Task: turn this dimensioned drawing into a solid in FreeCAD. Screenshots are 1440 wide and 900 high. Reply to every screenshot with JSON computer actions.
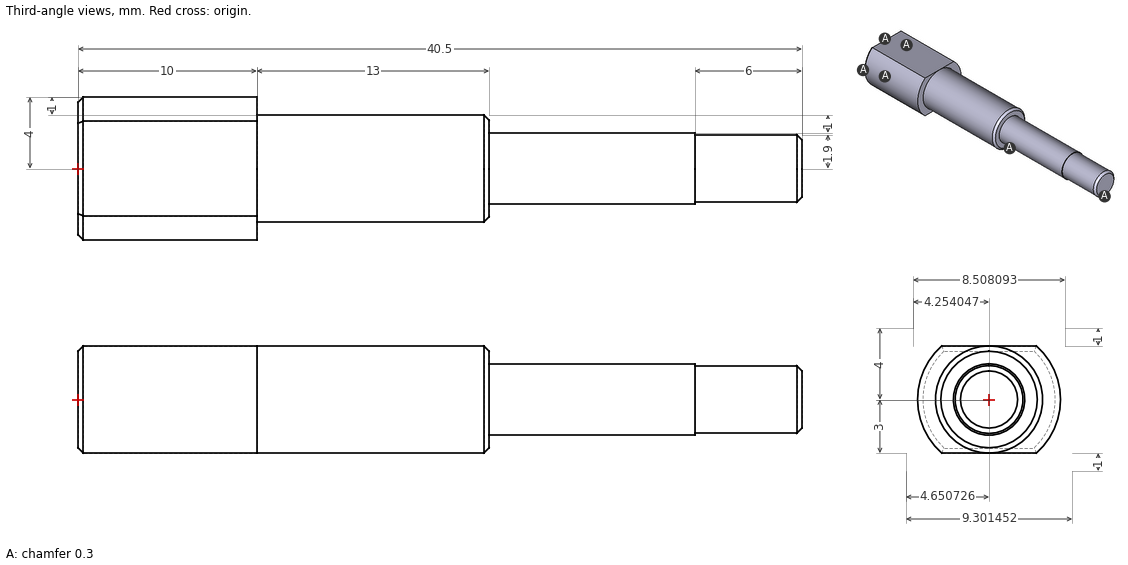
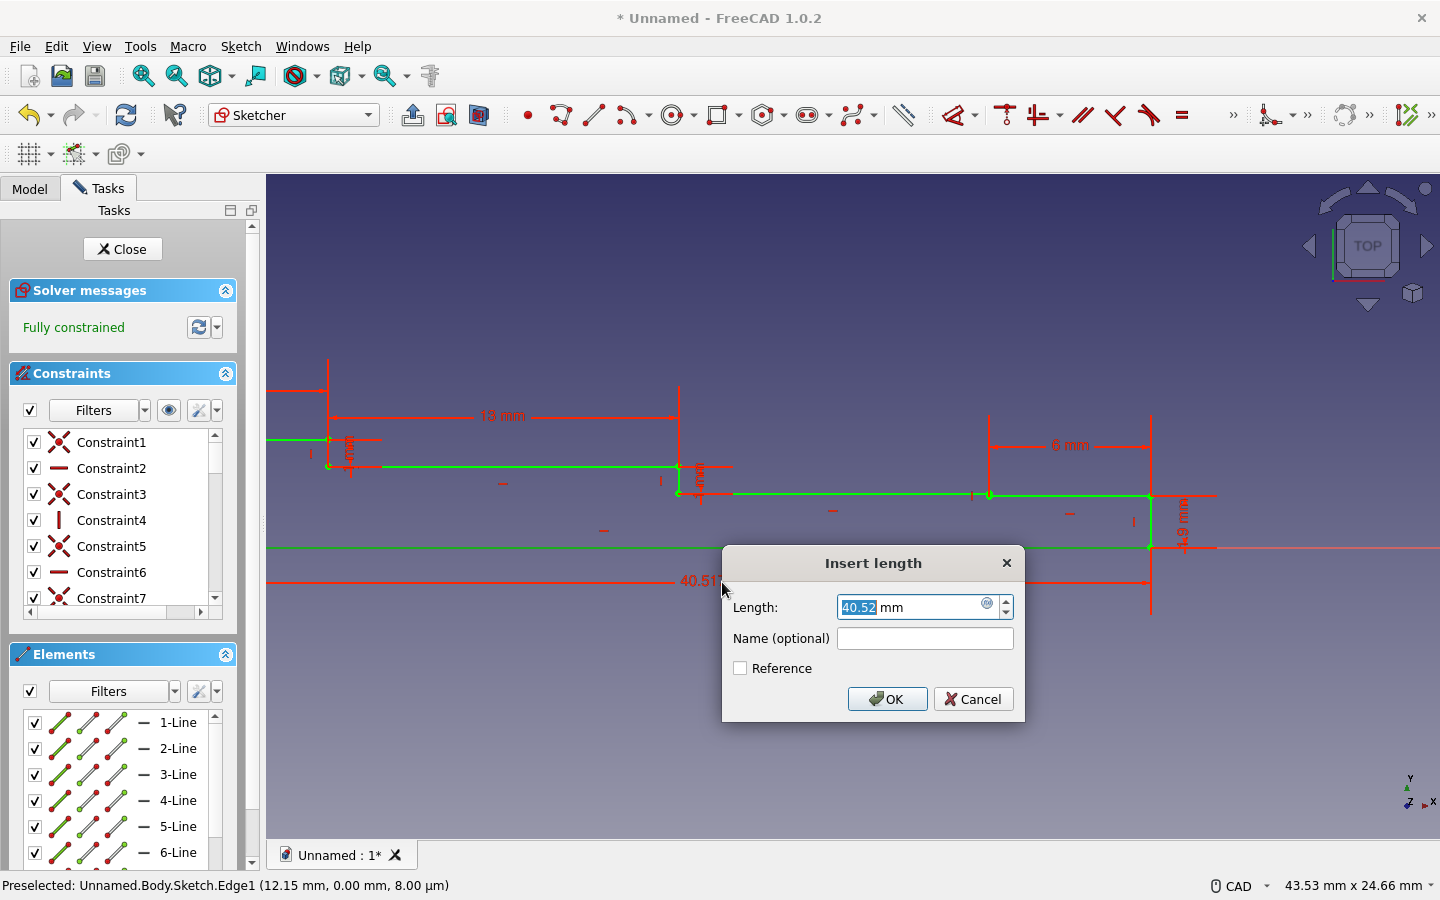
{"action": "type", "text": "40.5"}
{"action": "key", "text": "Return"}
{"action": "key", "text": "Escape"}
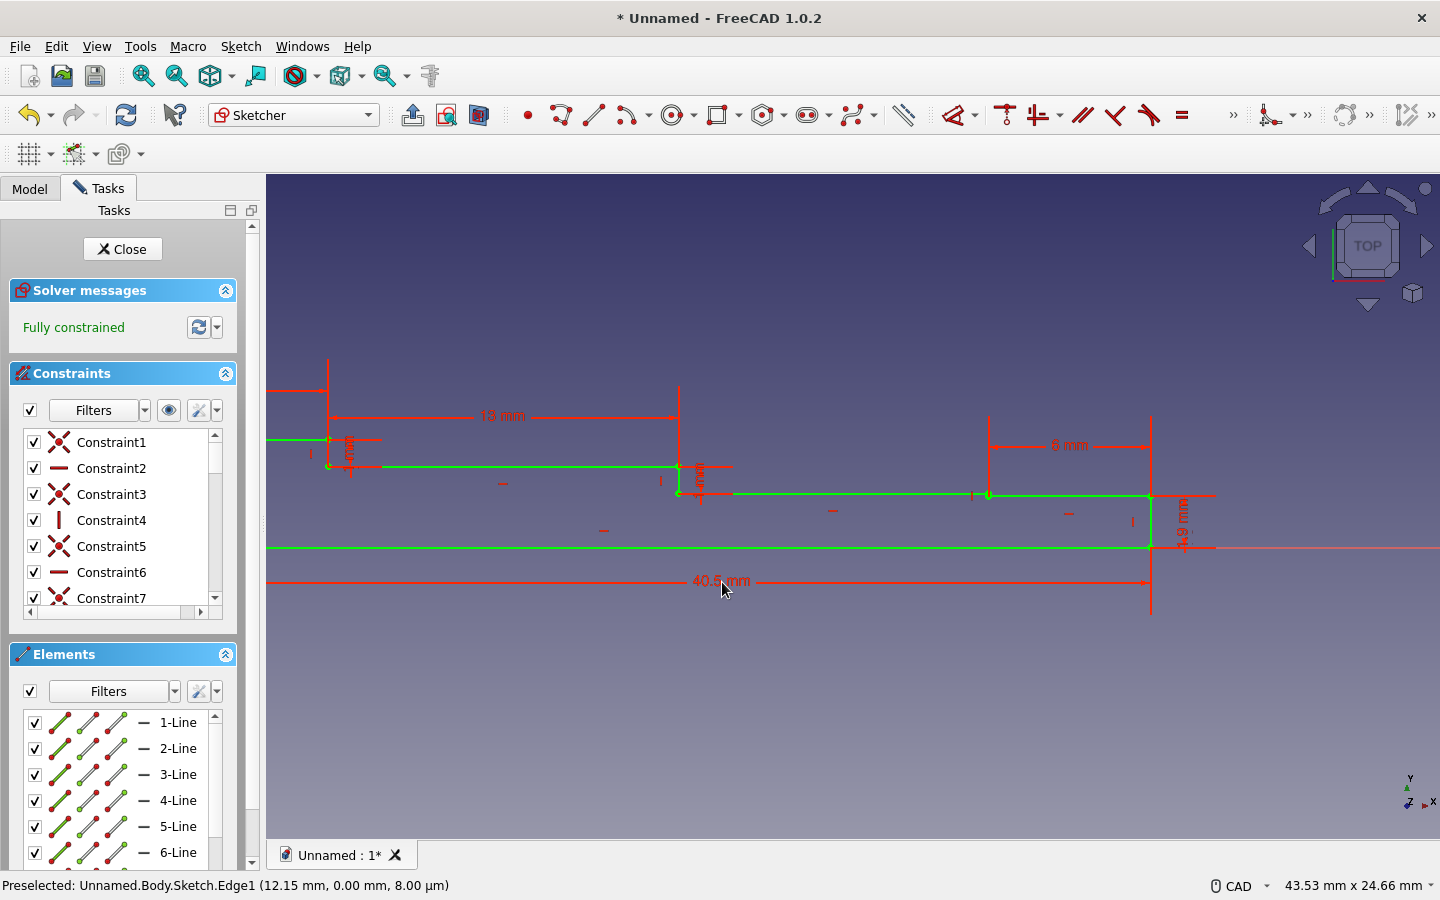
{"action": "left_click", "coordinate": [123, 249]}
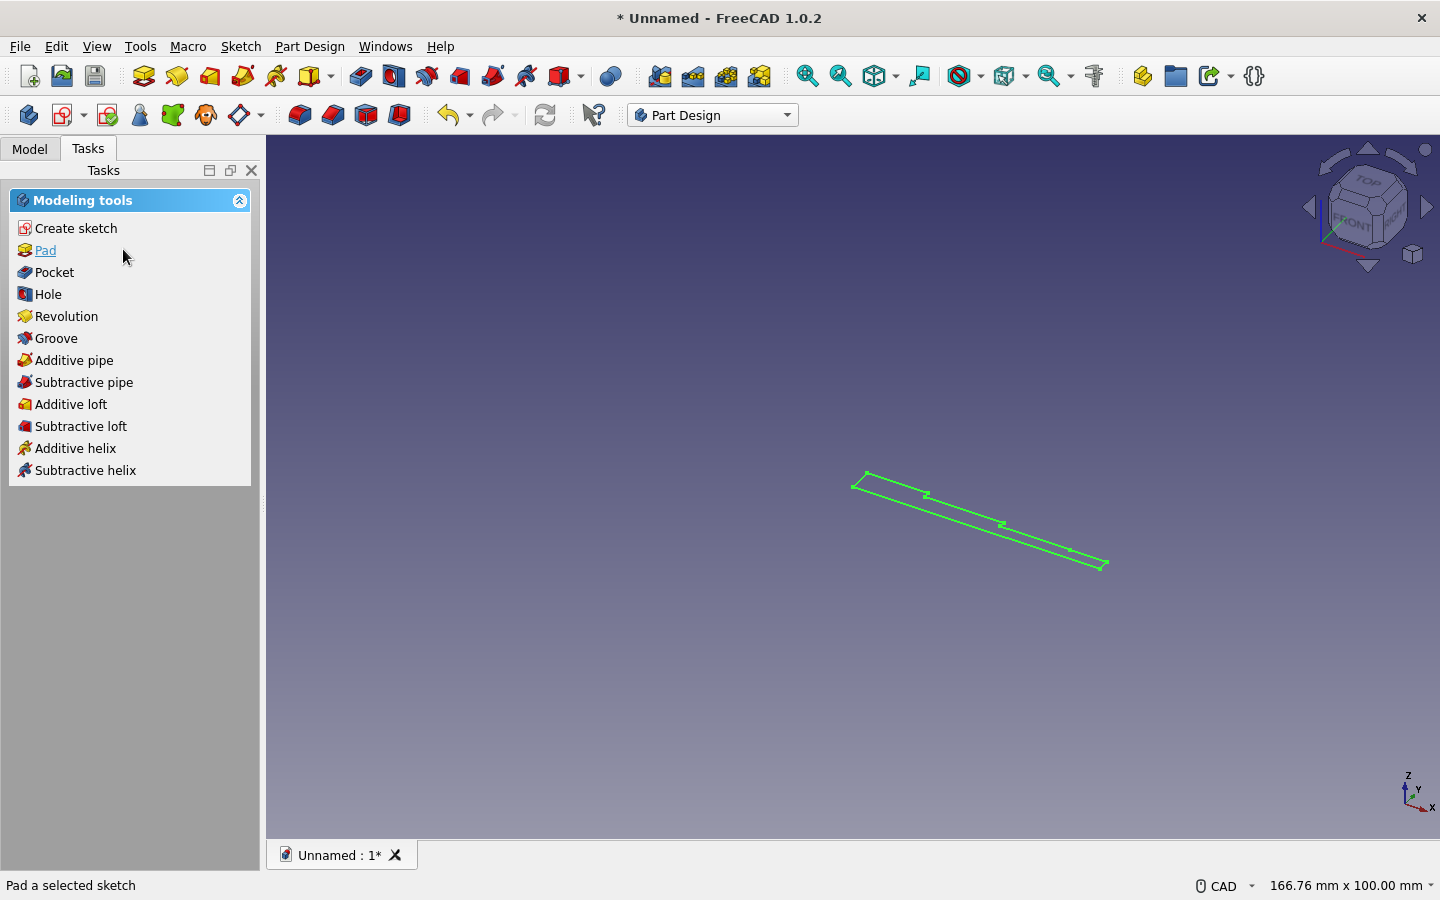
{"action": "left_click", "coordinate": [177, 76]}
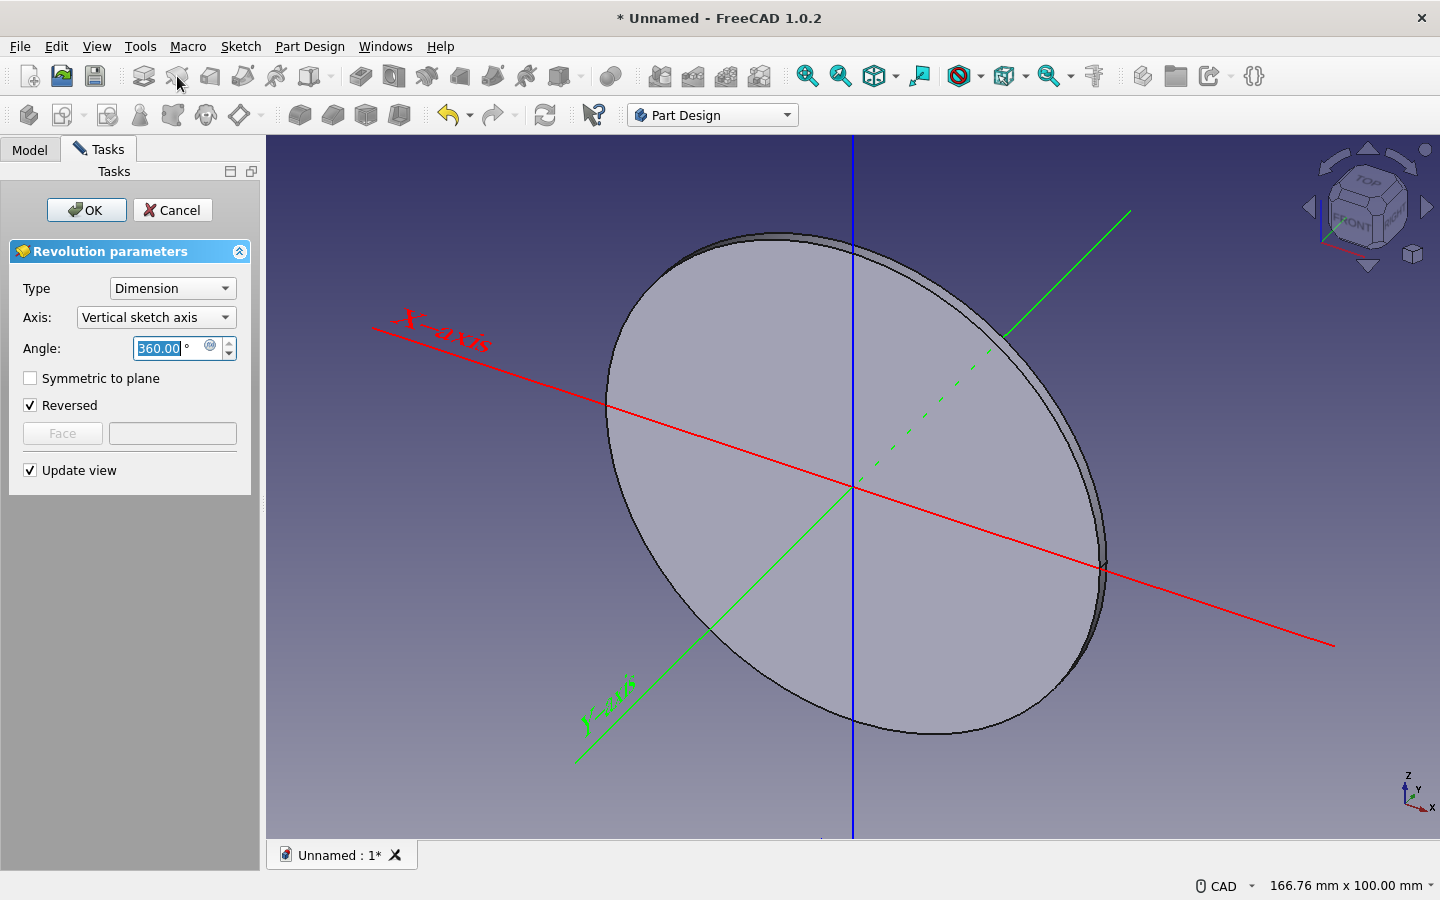
{"action": "left_click", "coordinate": [157, 318]}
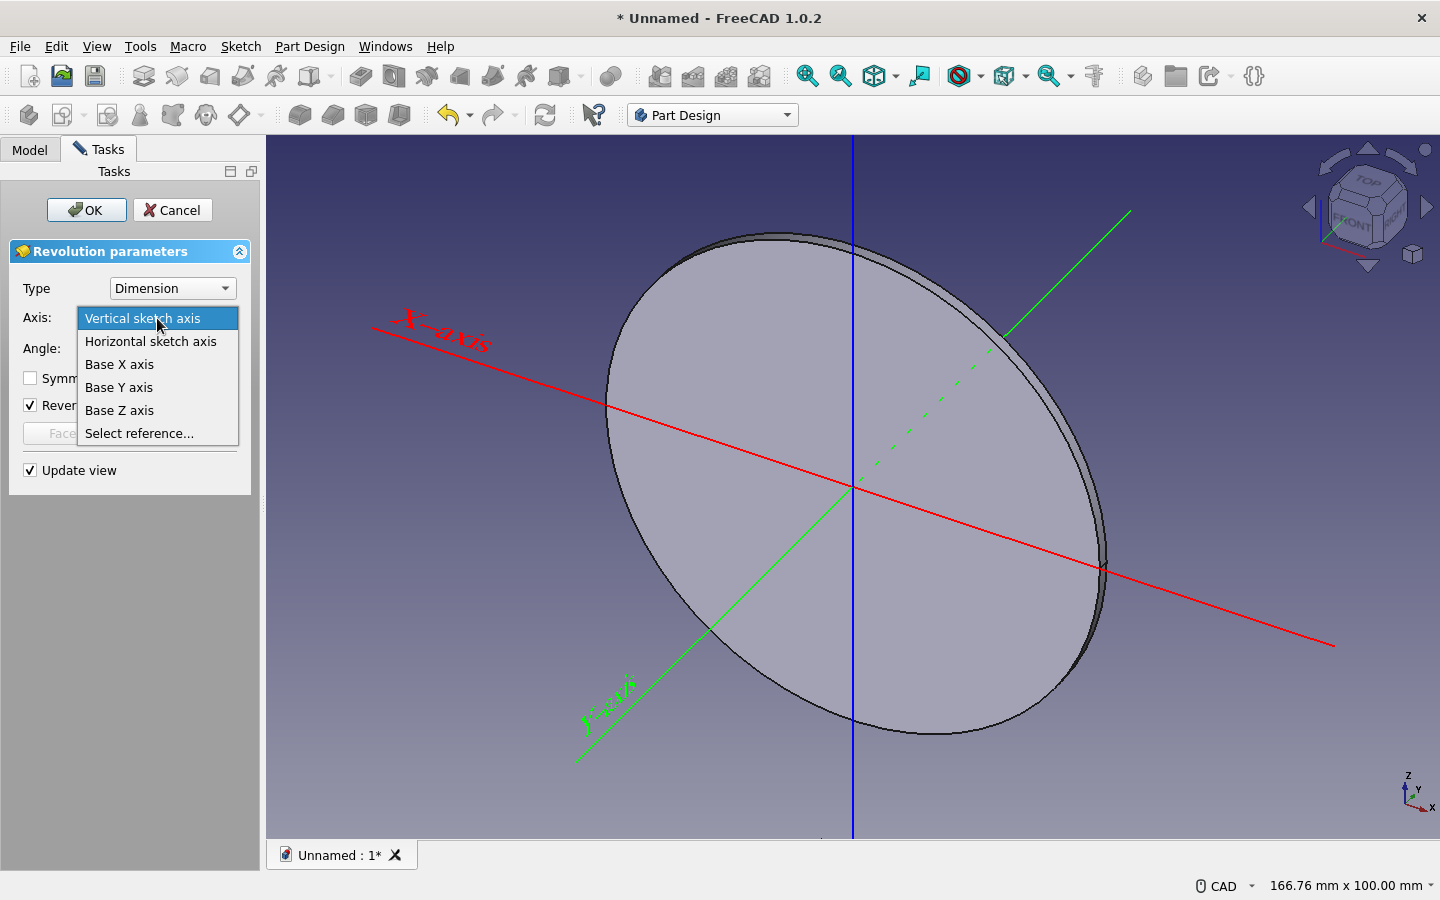
{"action": "left_click", "coordinate": [156, 342]}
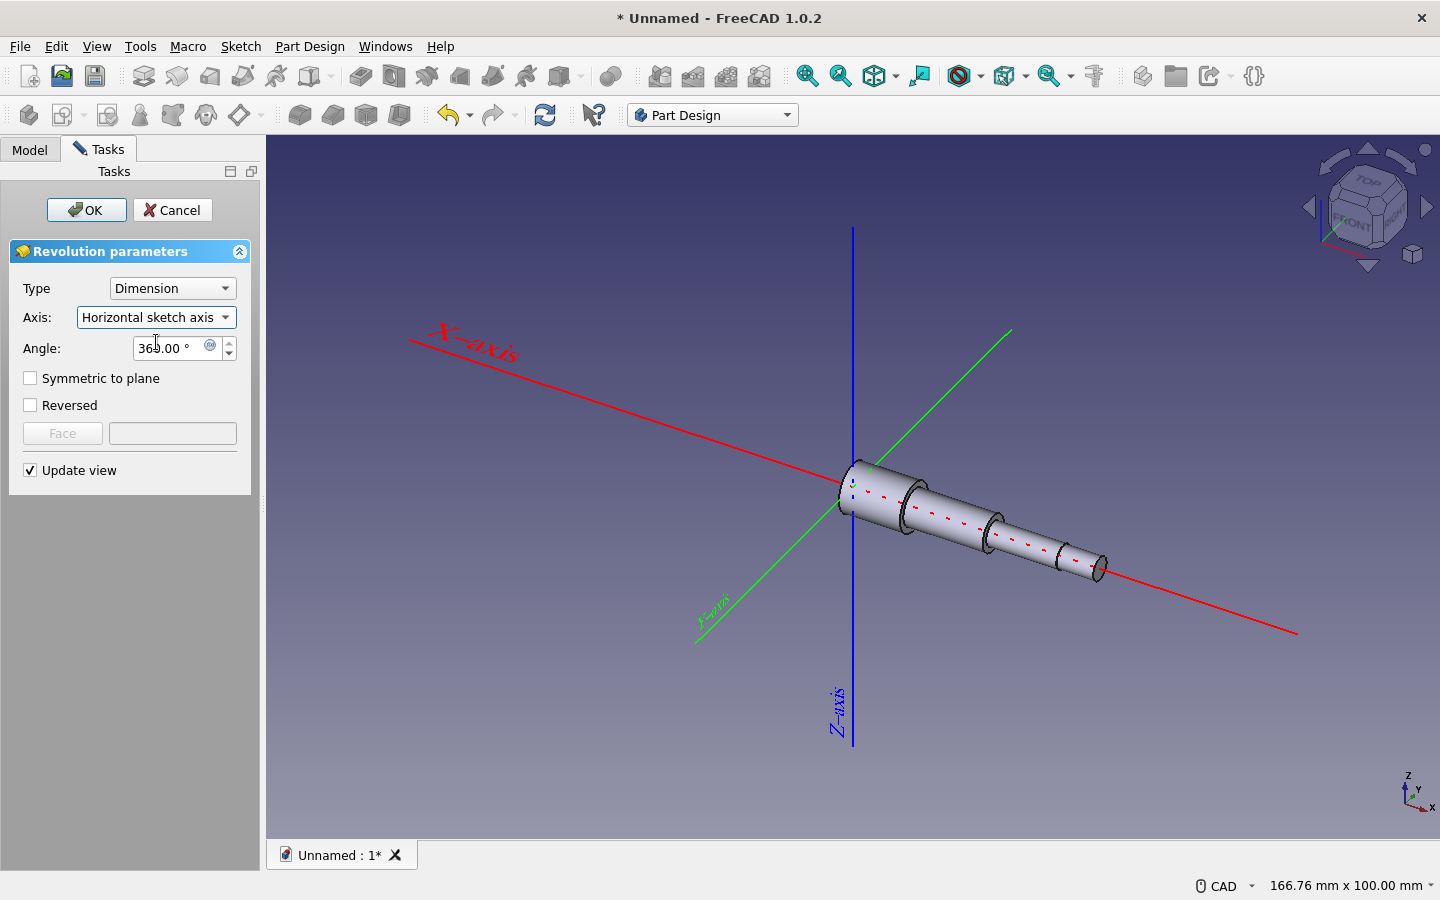
{"action": "left_click", "coordinate": [87, 210]}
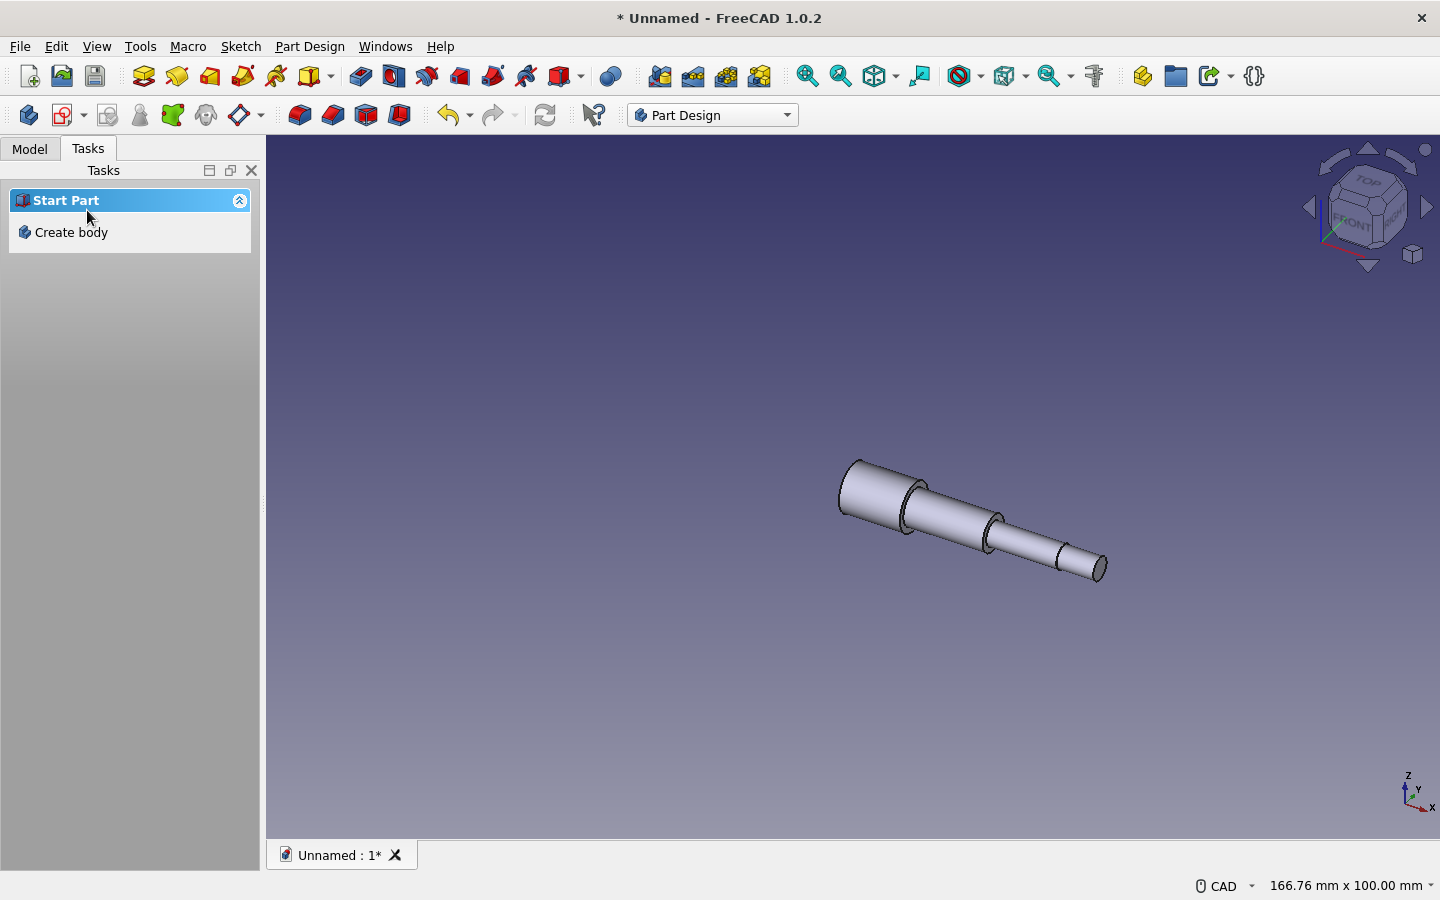
{"action": "left_click", "coordinate": [808, 76]}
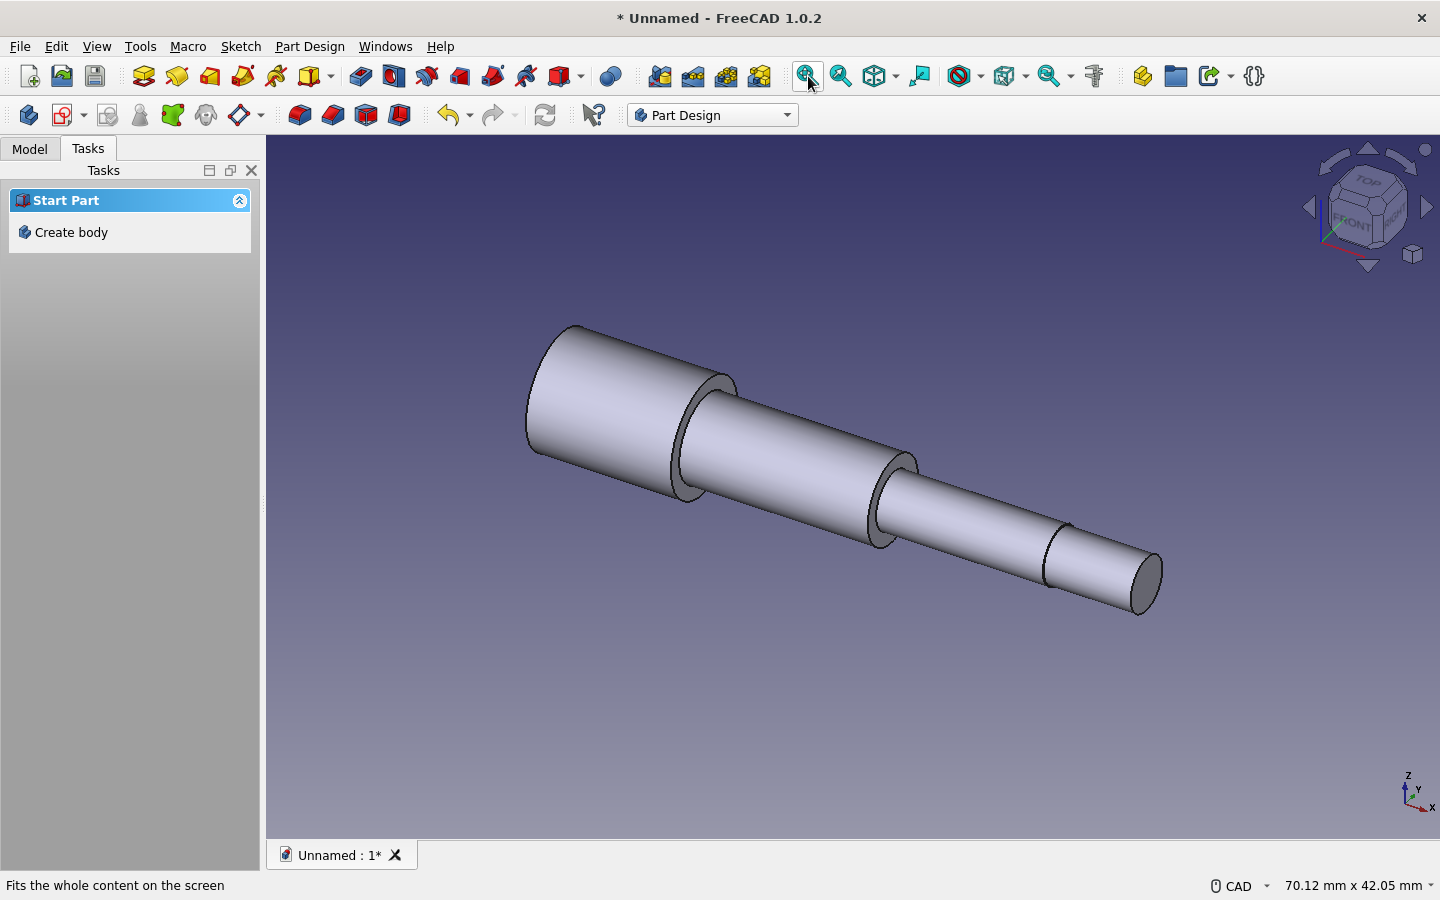
{"action": "left_click", "coordinate": [62, 116]}